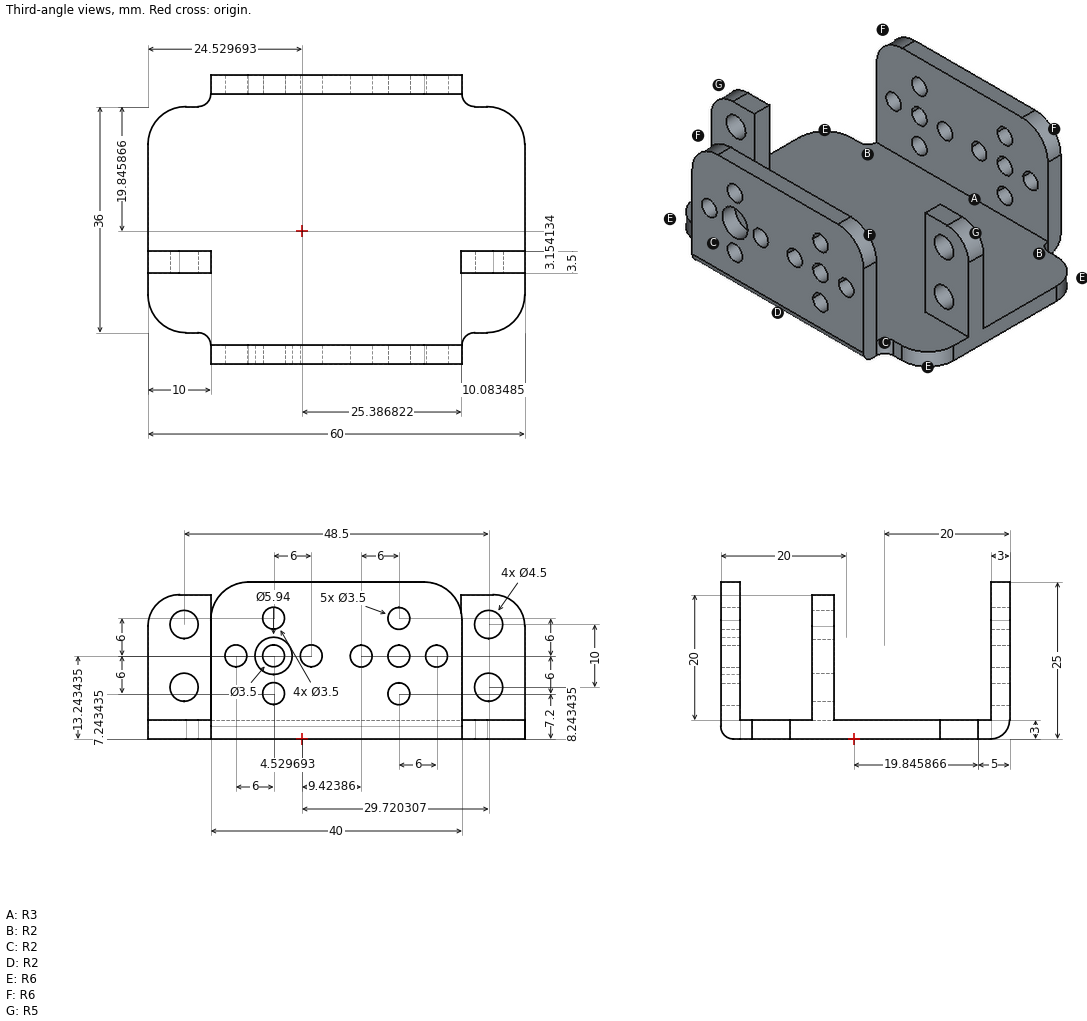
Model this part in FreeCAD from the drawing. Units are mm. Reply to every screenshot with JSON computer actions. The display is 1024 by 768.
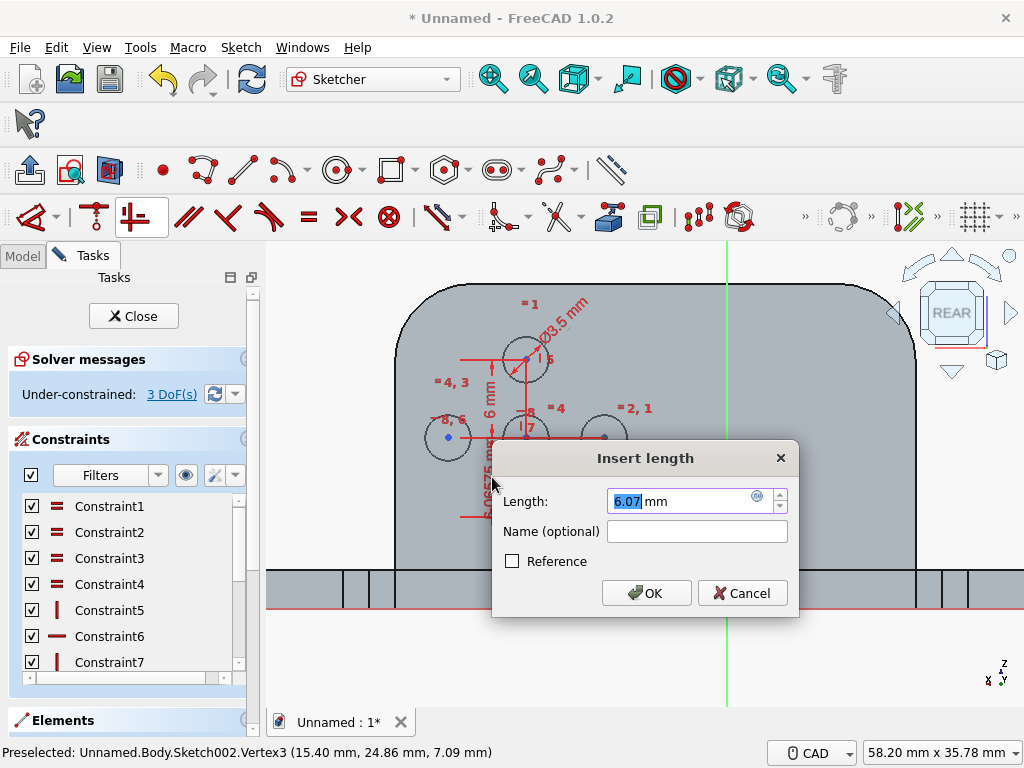
{"action": "type", "text": "6"}
{"action": "key", "text": "Return"}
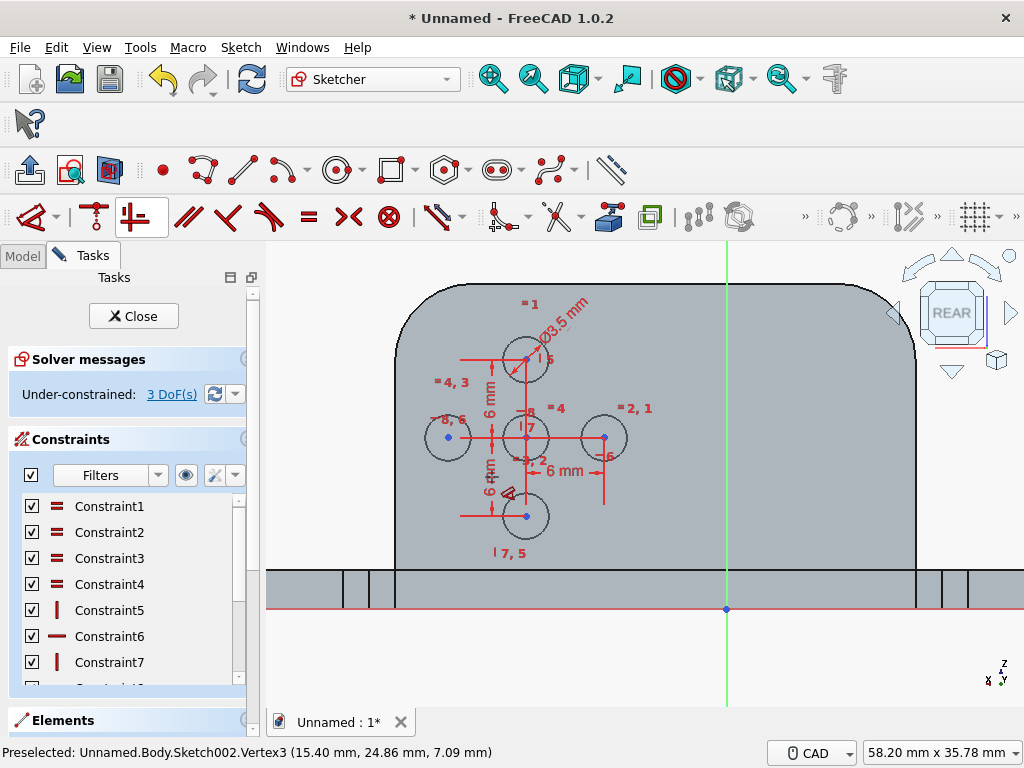
{"action": "left_click", "coordinate": [526, 516]}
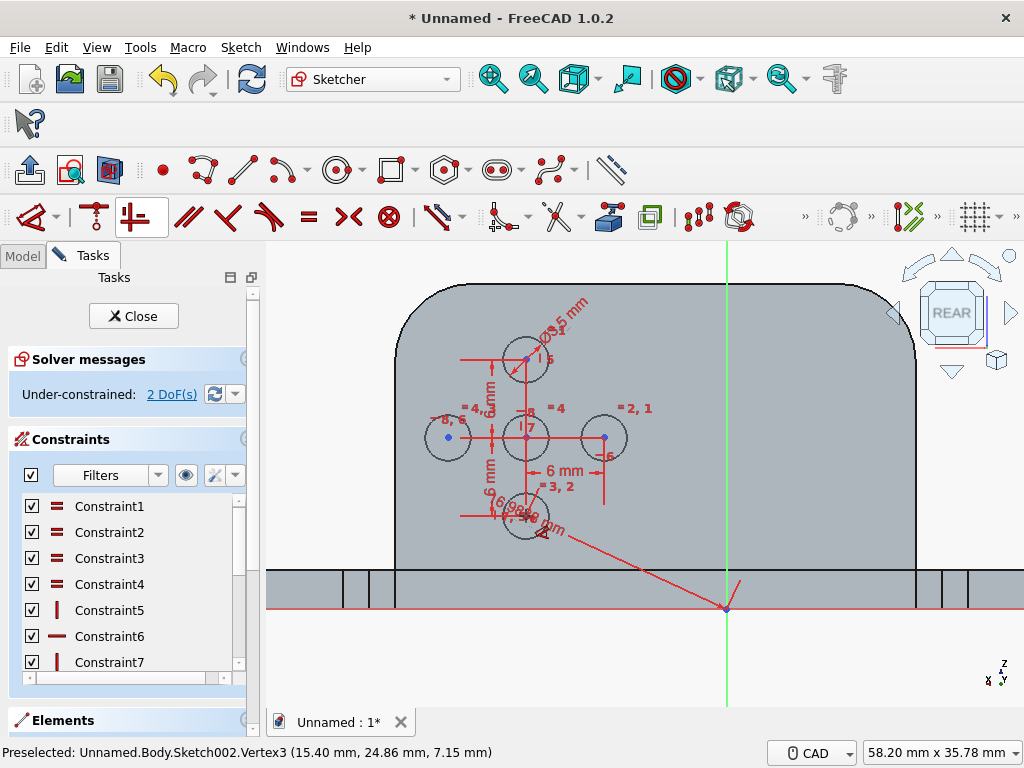
{"action": "left_click", "coordinate": [448, 438]}
{"action": "left_click", "coordinate": [487, 550]}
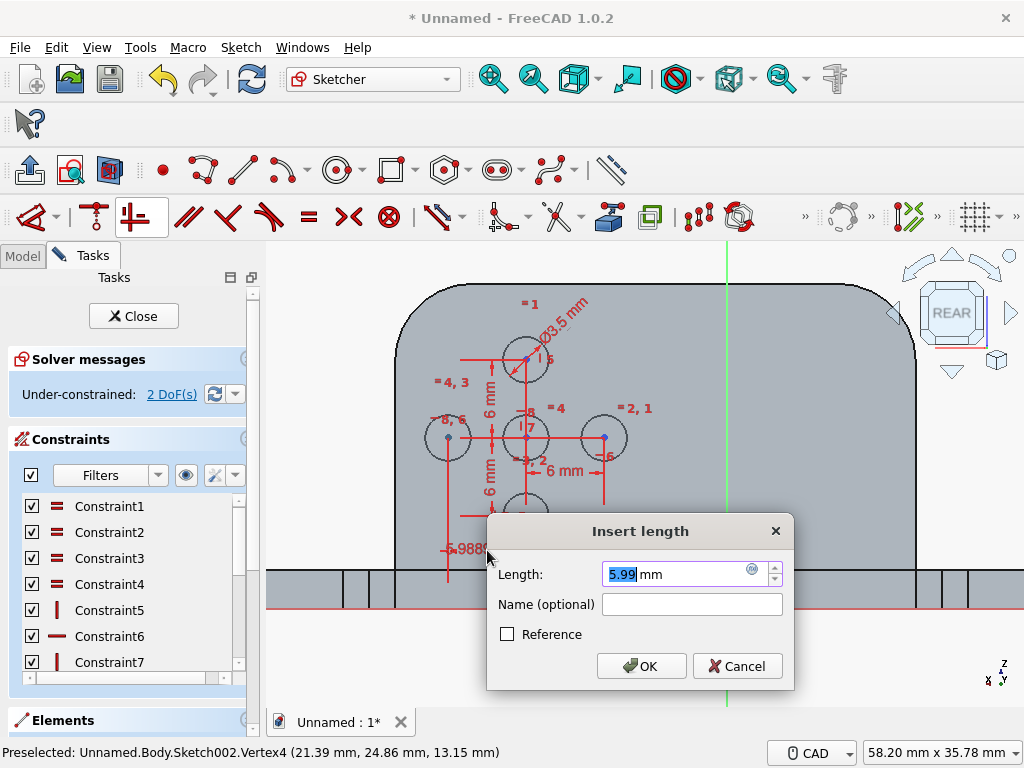
{"action": "type", "text": "6"}
{"action": "key", "text": "Return"}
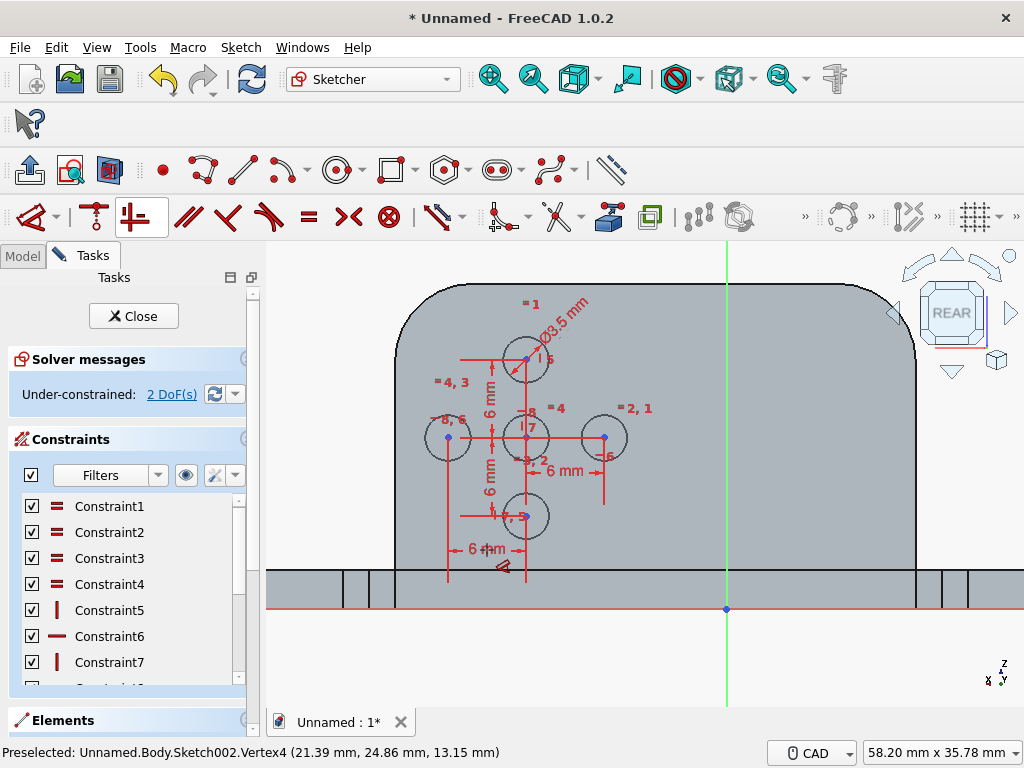
{"action": "left_click", "coordinate": [526, 516]}
{"action": "left_click", "coordinate": [761, 563]}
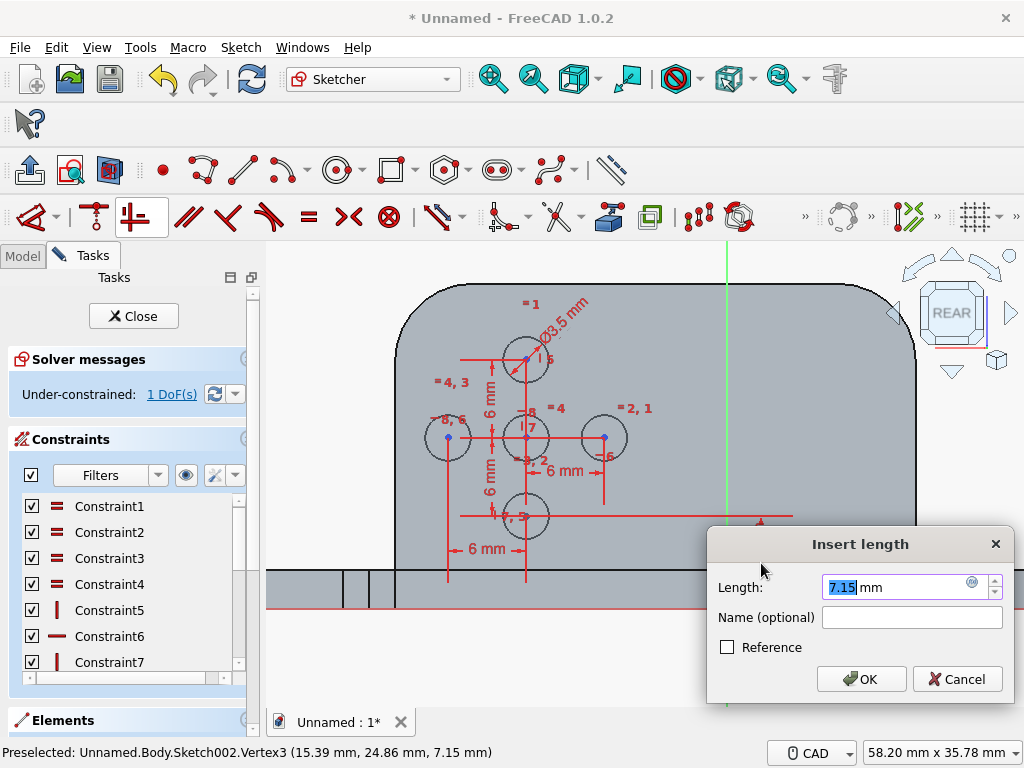
{"action": "type", "text": "7.2"}
{"action": "key", "text": "Return"}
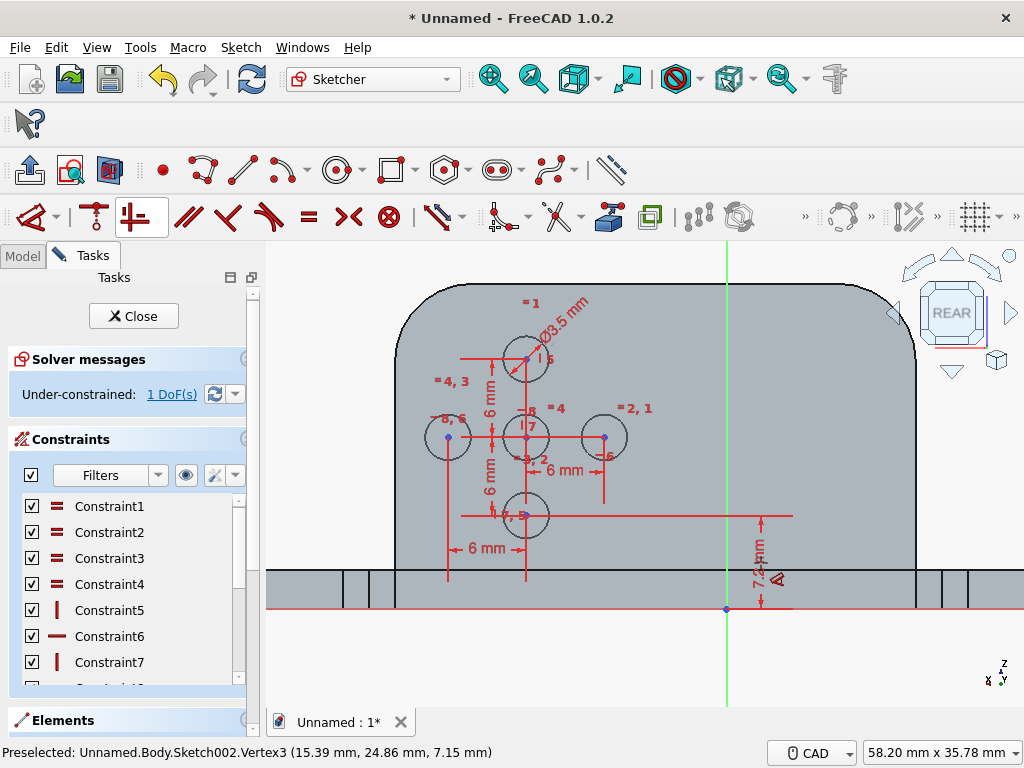
{"action": "left_click", "coordinate": [604, 437]}
{"action": "left_click", "coordinate": [665, 643]}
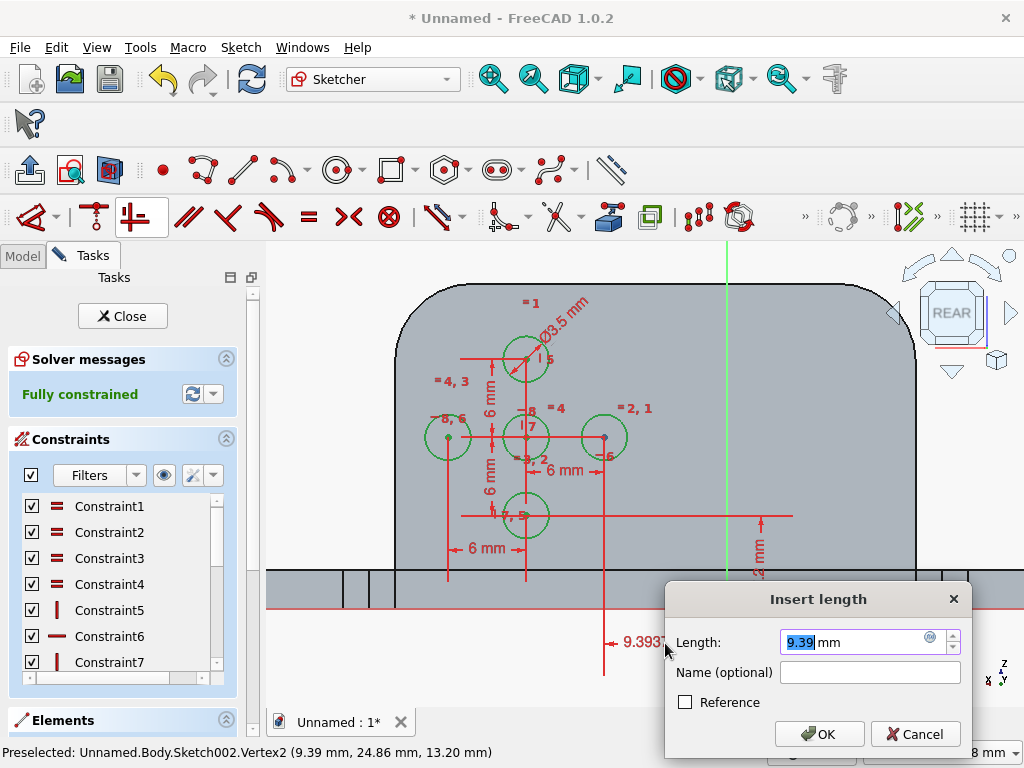
{"action": "type", "text": "9.42386"}
{"action": "key", "text": "Return"}
{"action": "key", "text": "Escape"}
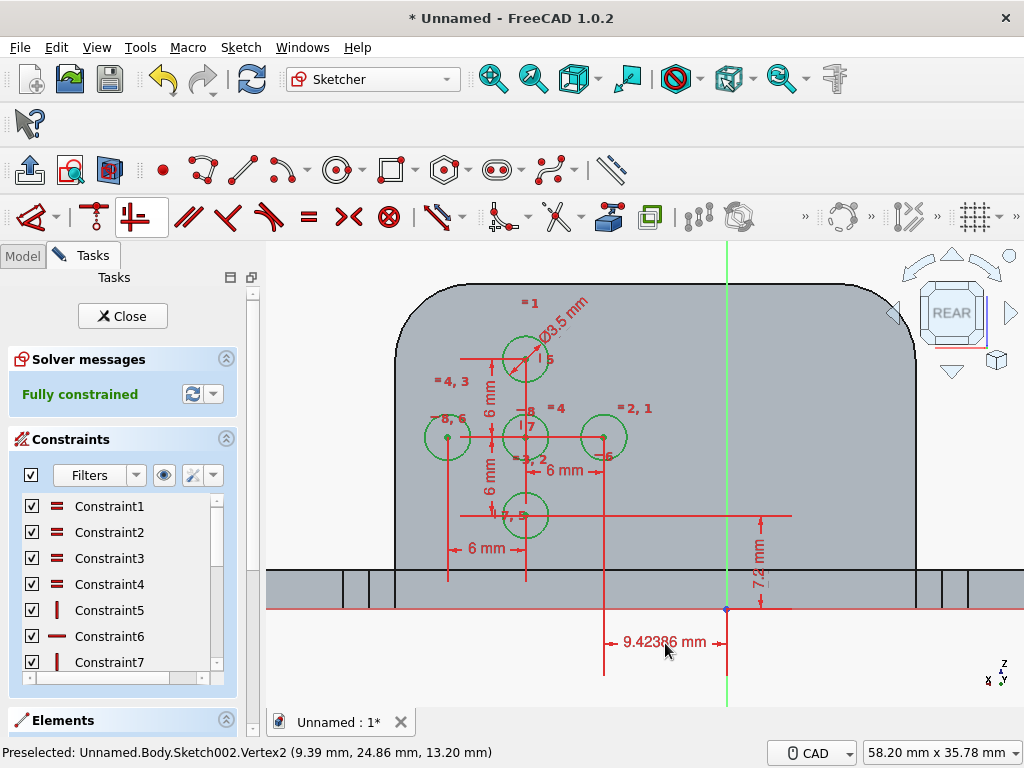
{"action": "left_click", "coordinate": [123, 316]}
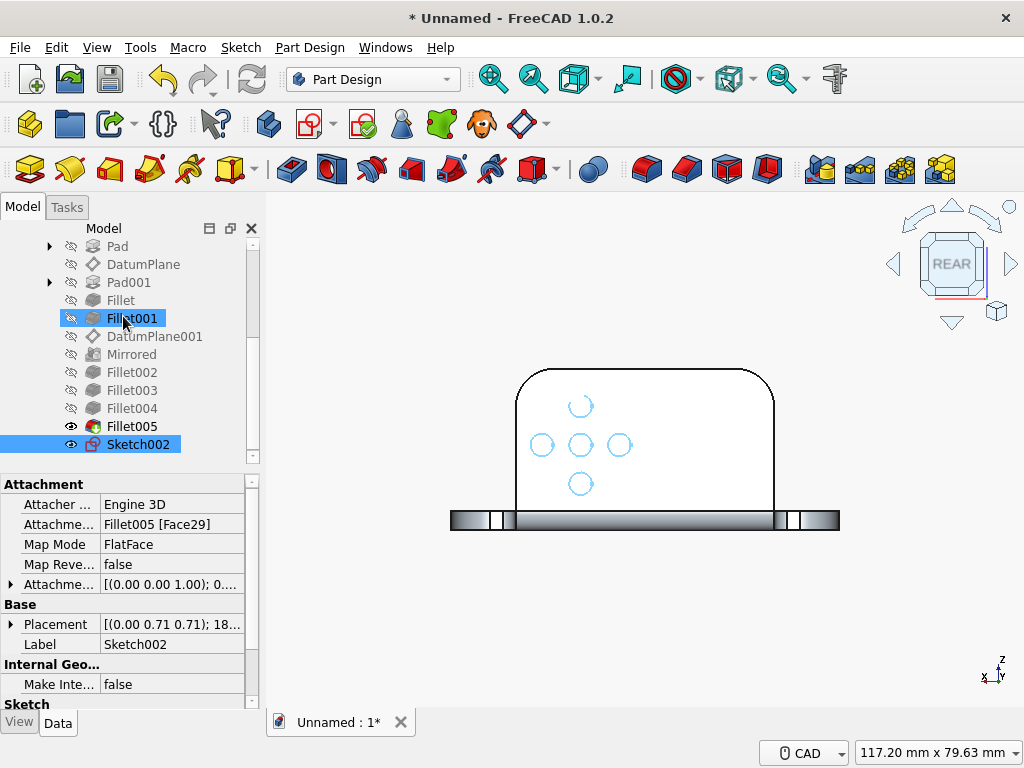
{"action": "left_click", "coordinate": [292, 170]}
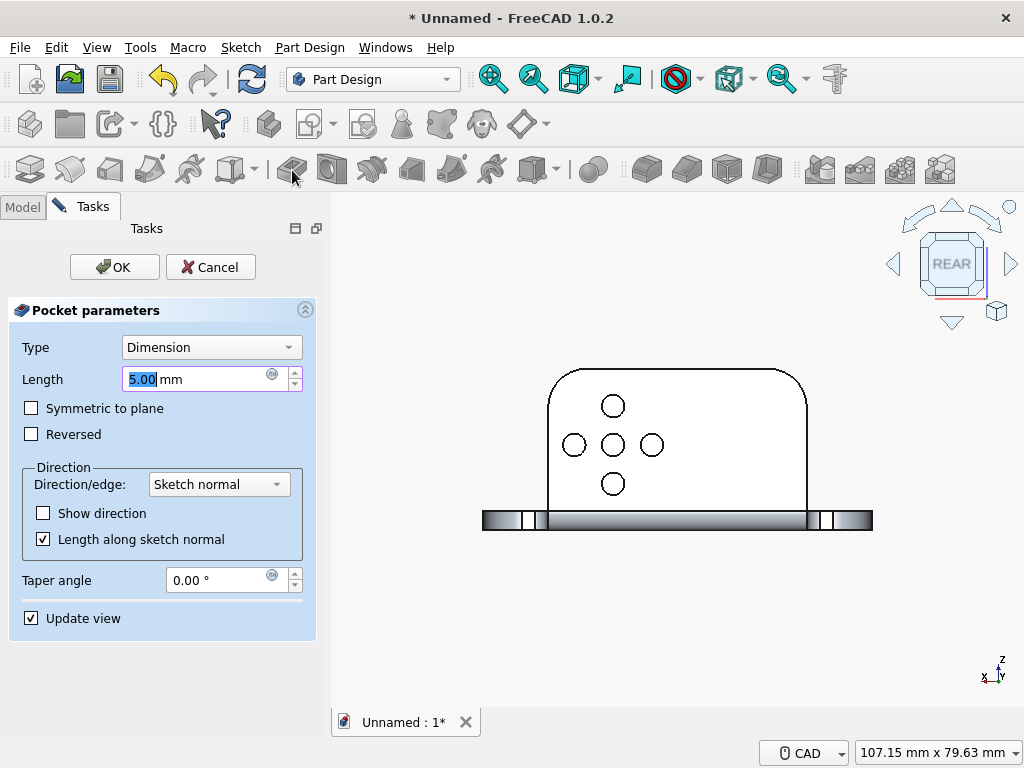
{"action": "left_click", "coordinate": [212, 348]}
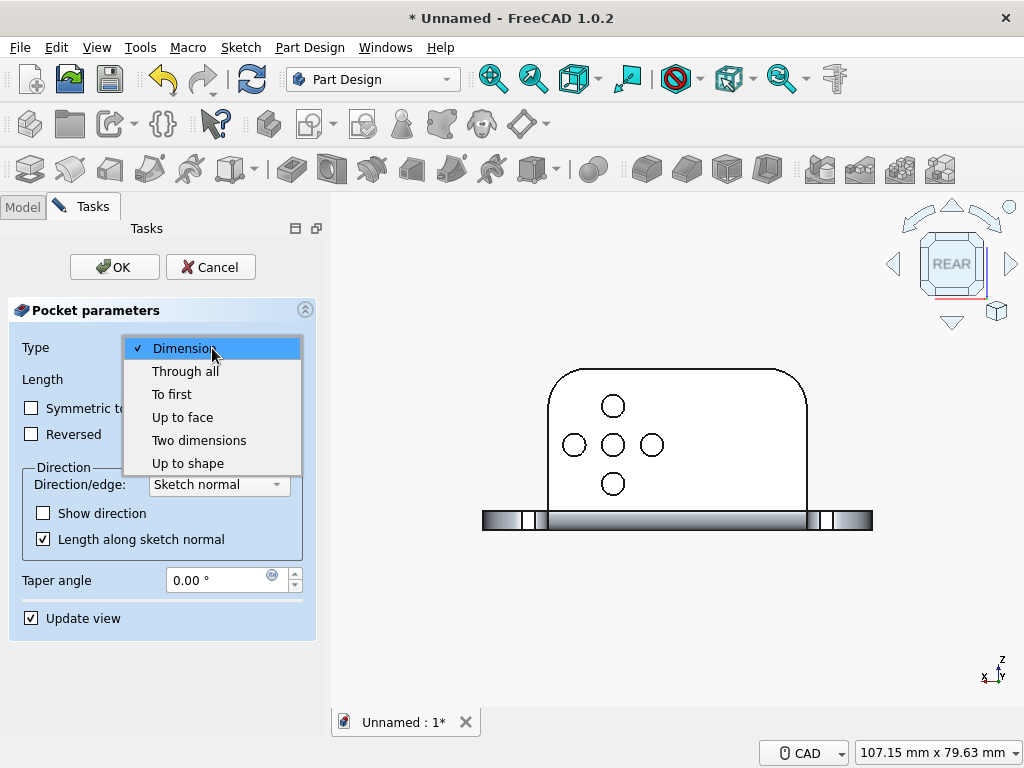
{"action": "left_click", "coordinate": [212, 372]}